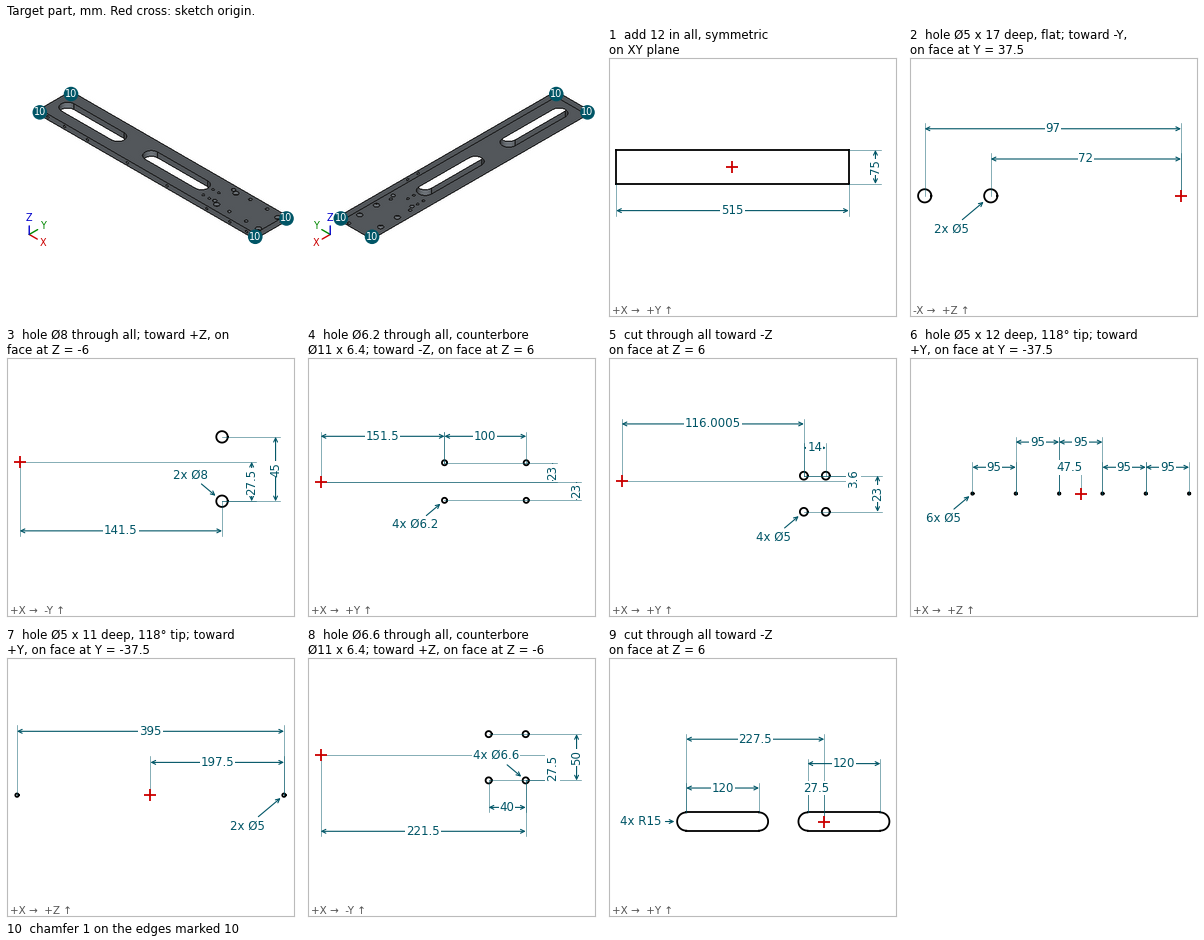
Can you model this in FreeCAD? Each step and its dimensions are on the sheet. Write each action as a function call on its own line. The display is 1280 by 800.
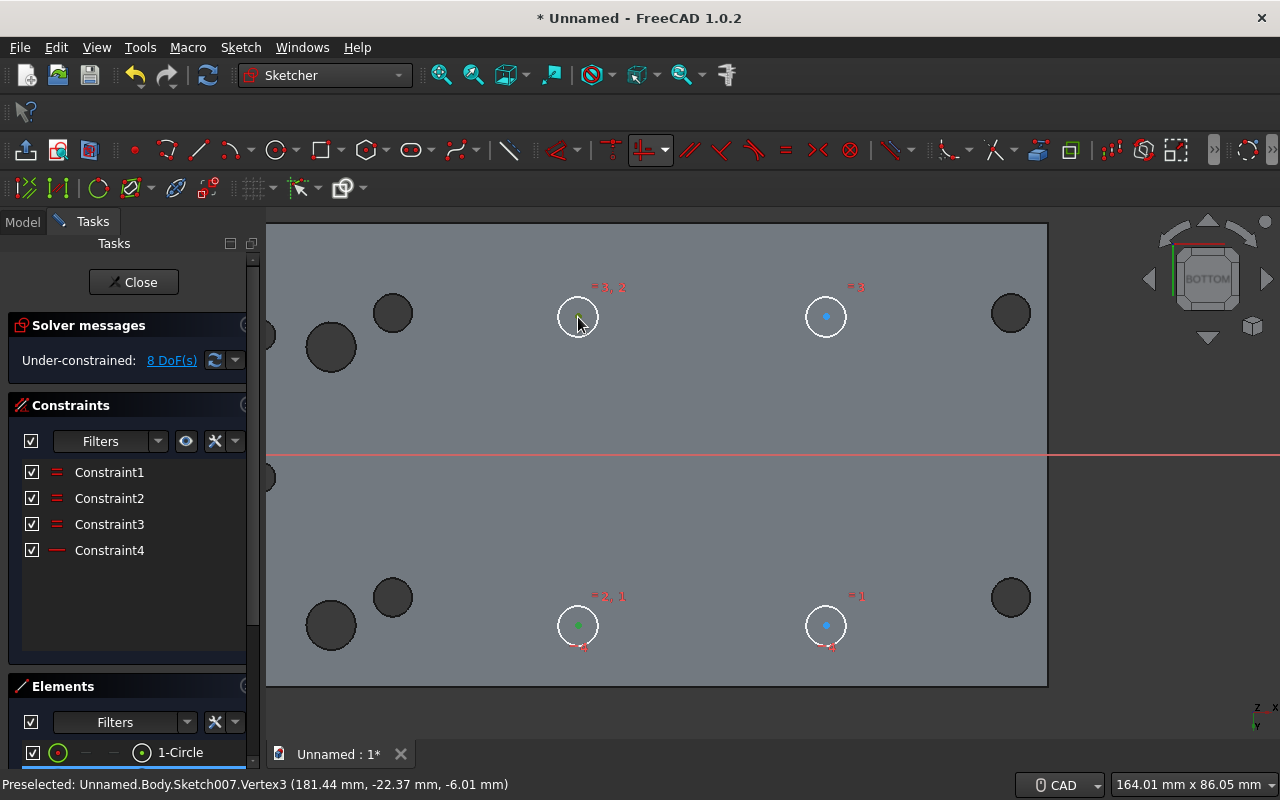
key(v)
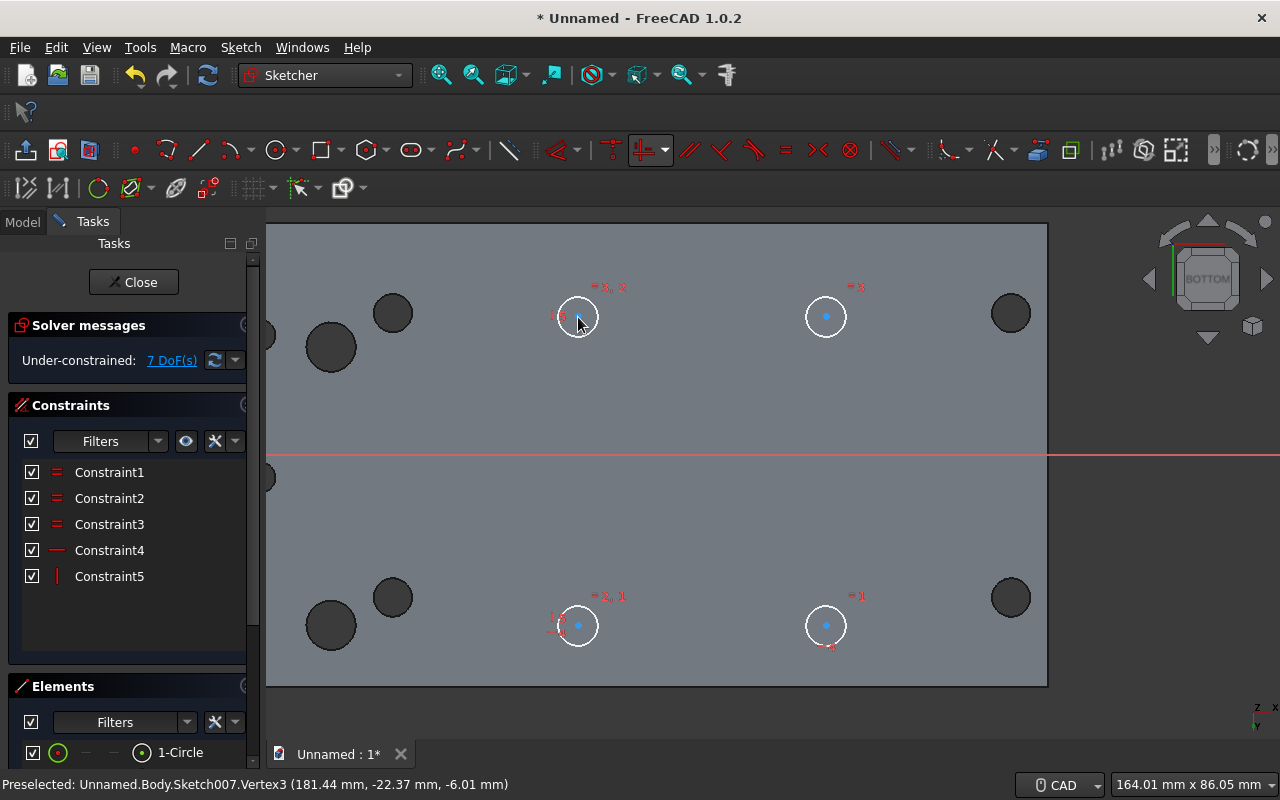
click(826, 626)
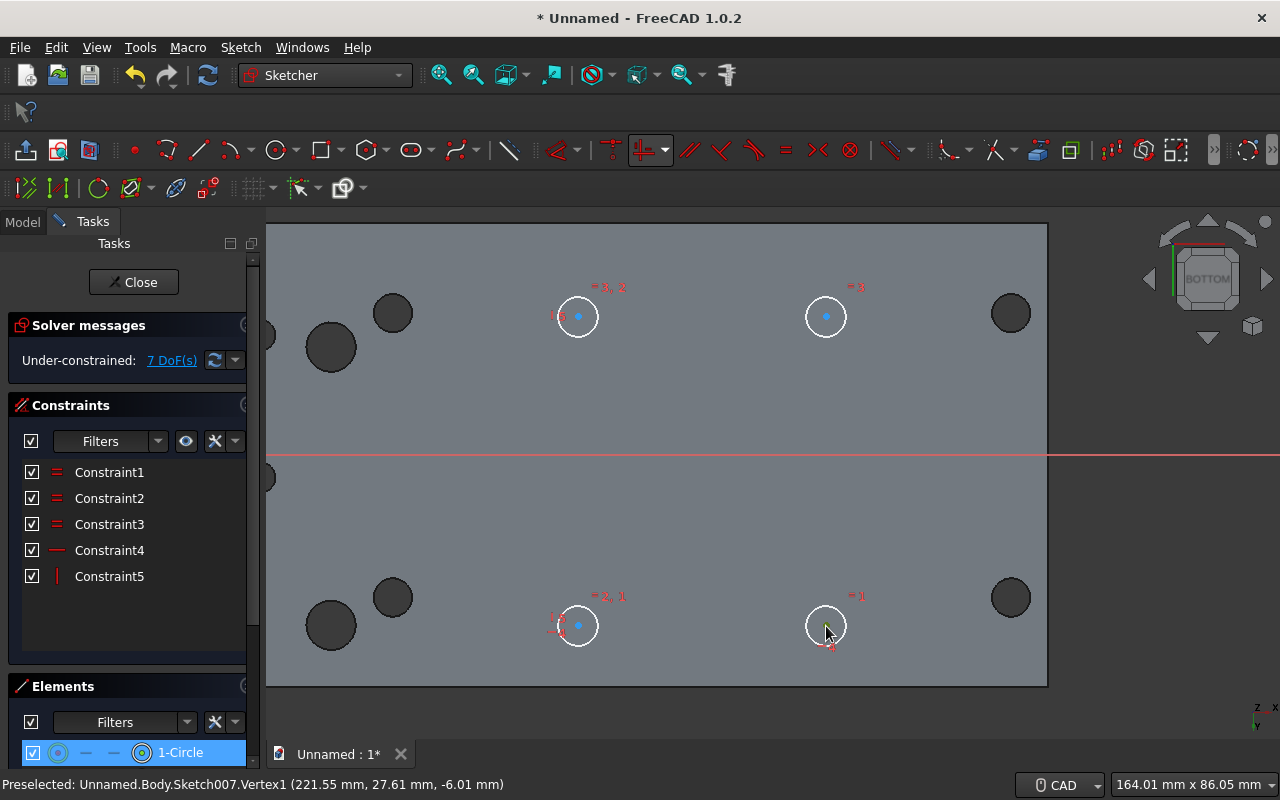
click(826, 317)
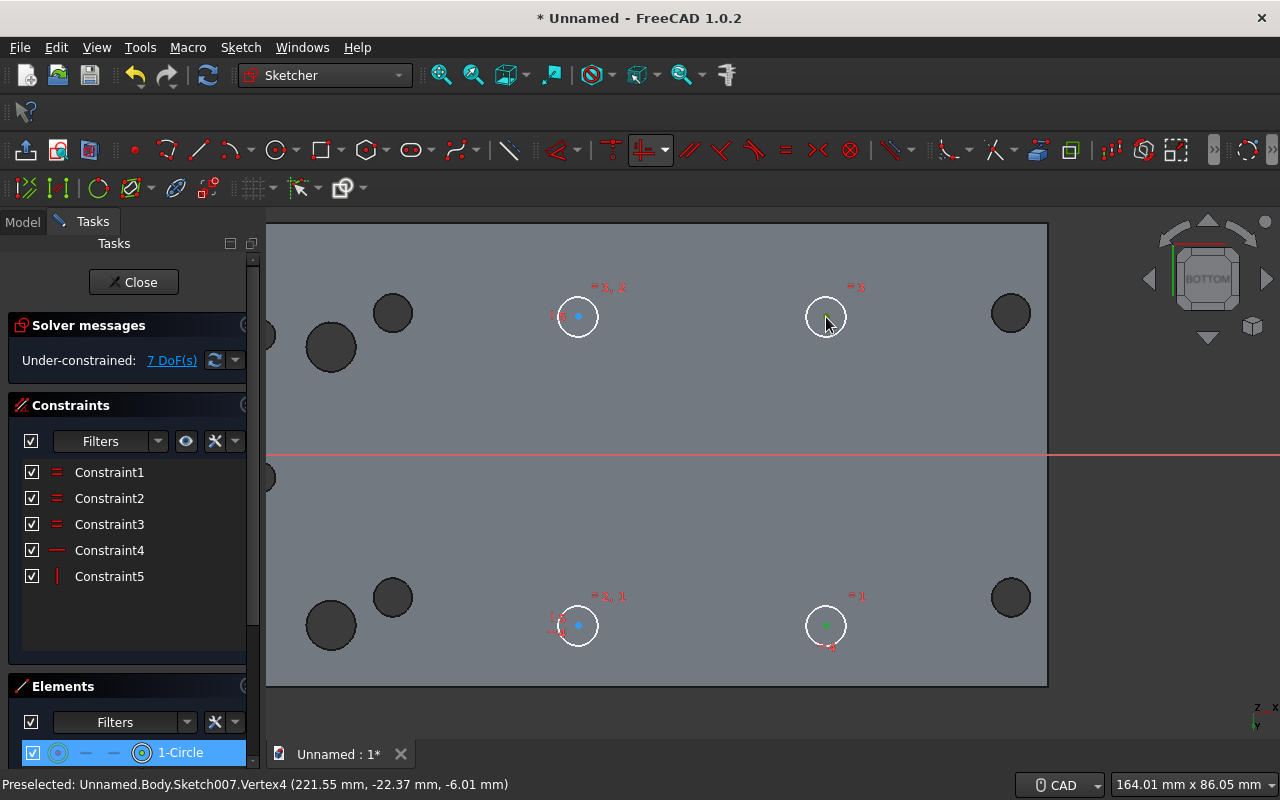
key(v)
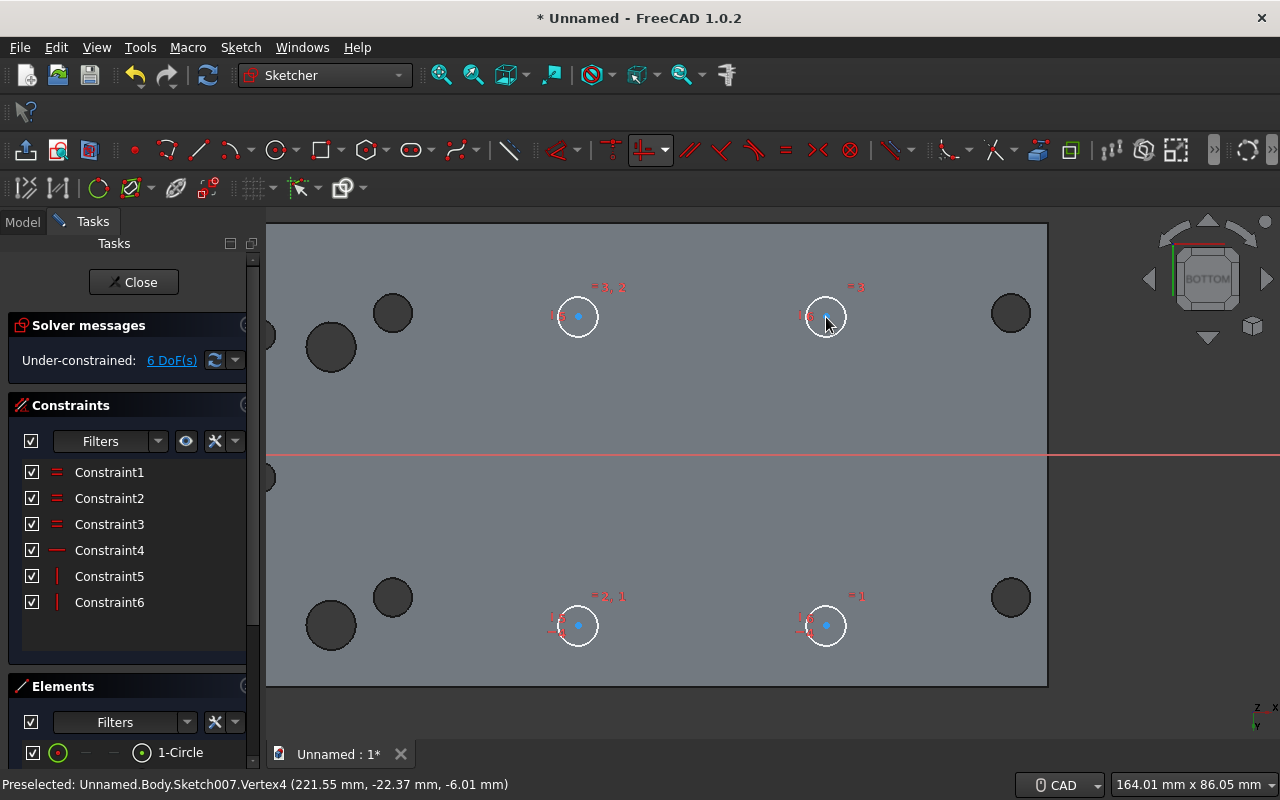
click(578, 317)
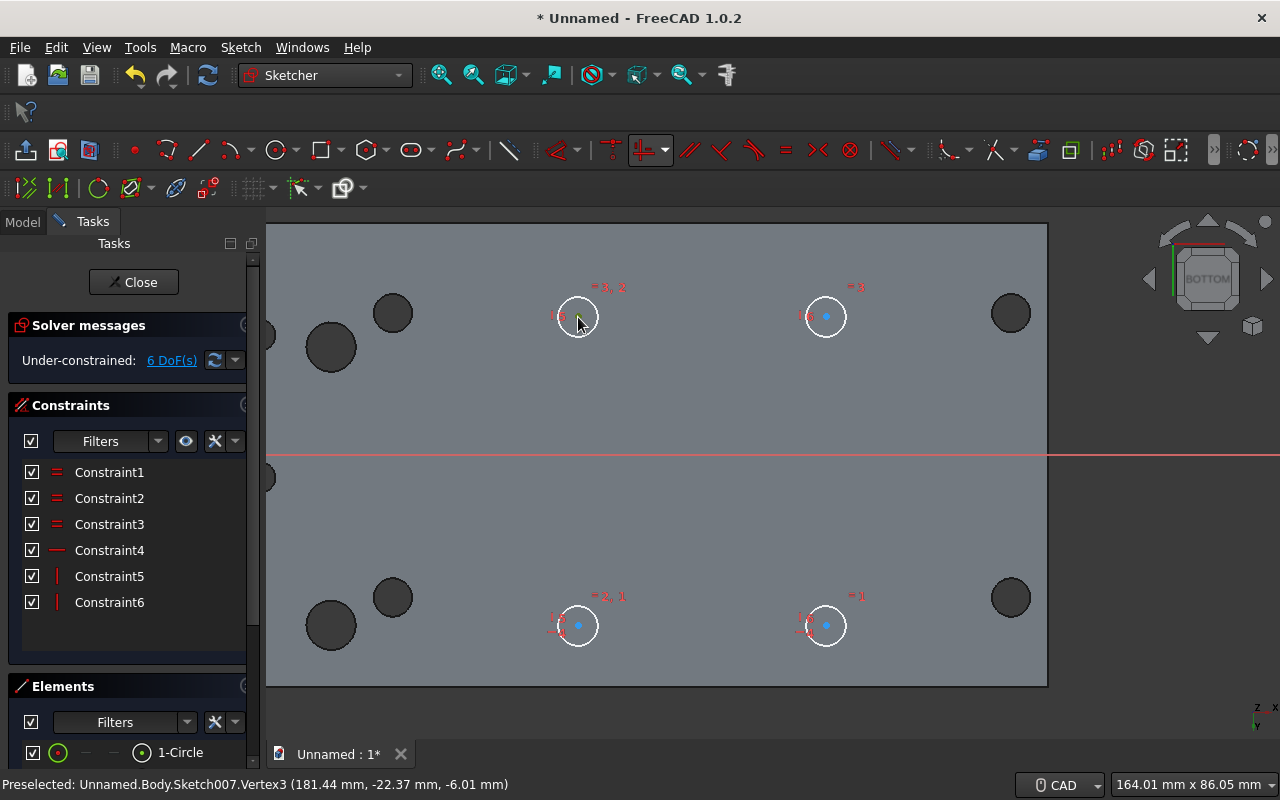
click(826, 317)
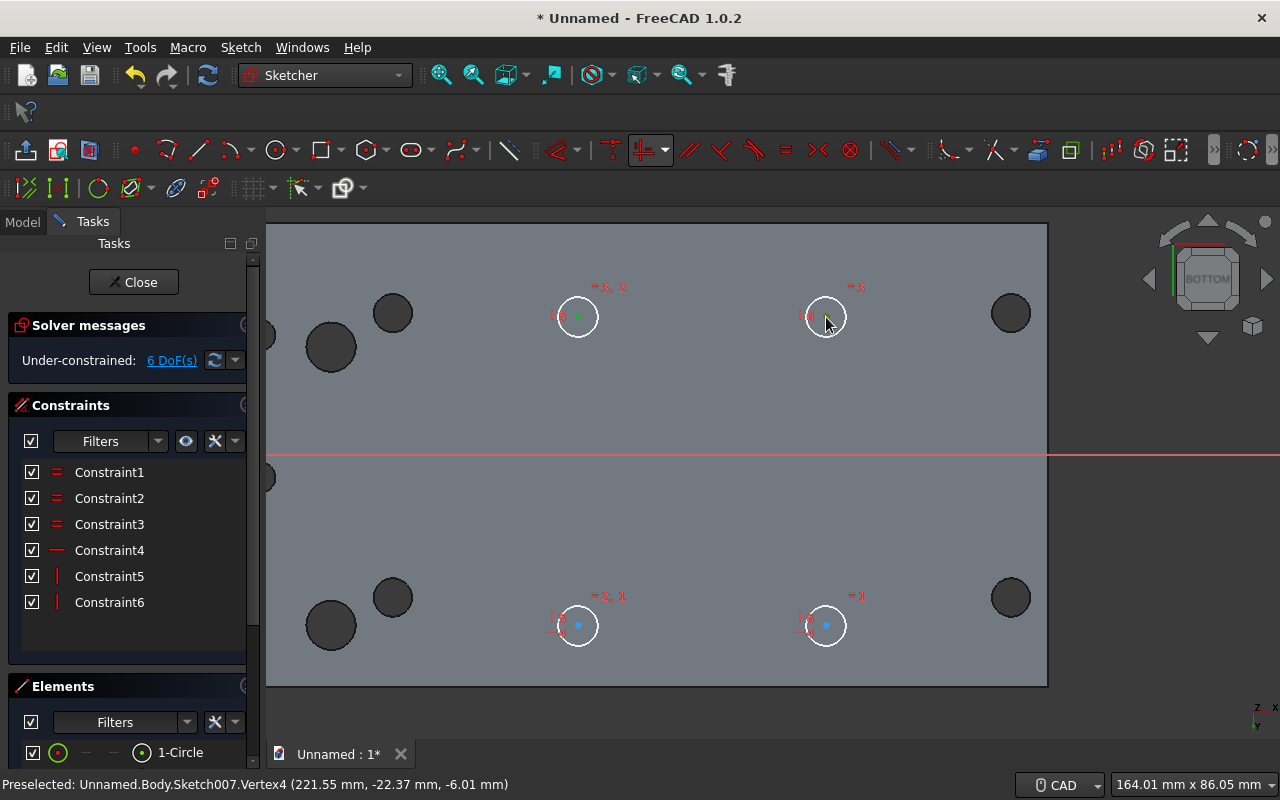
click(668, 150)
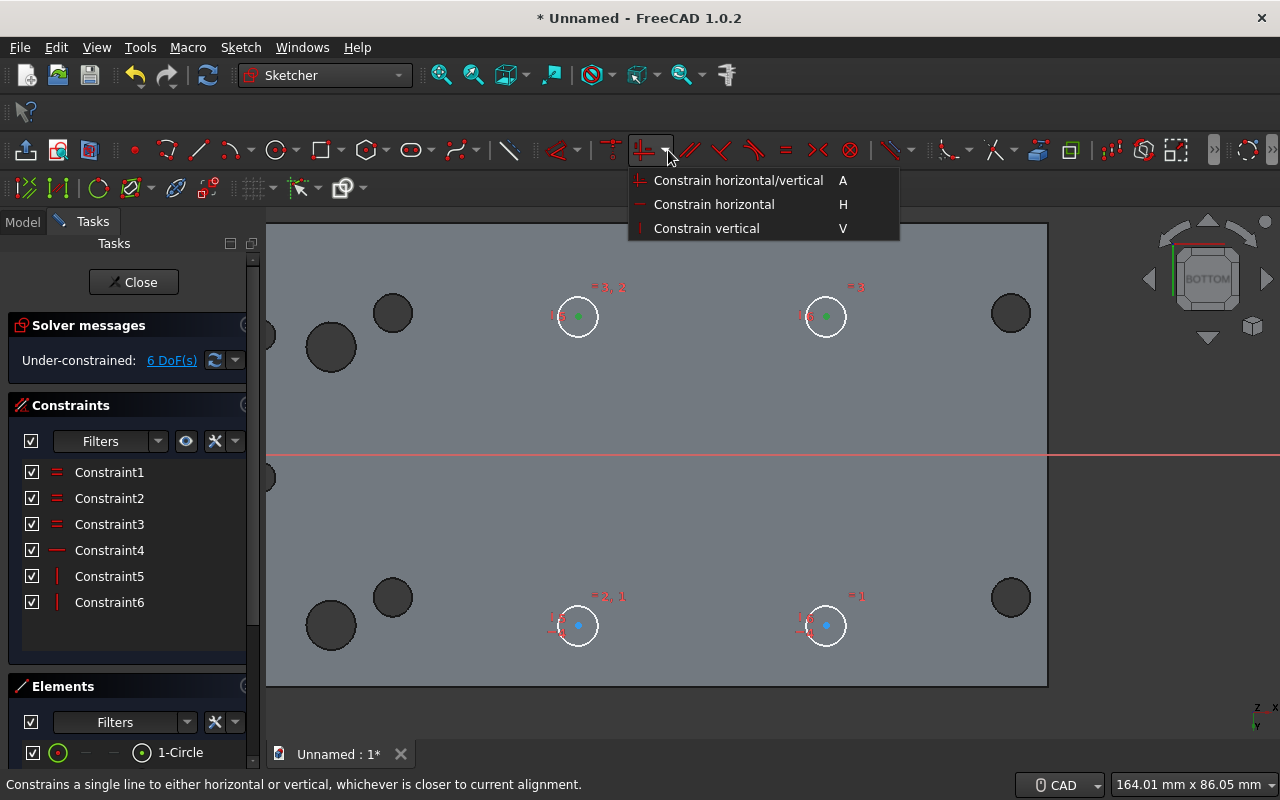
click(764, 204)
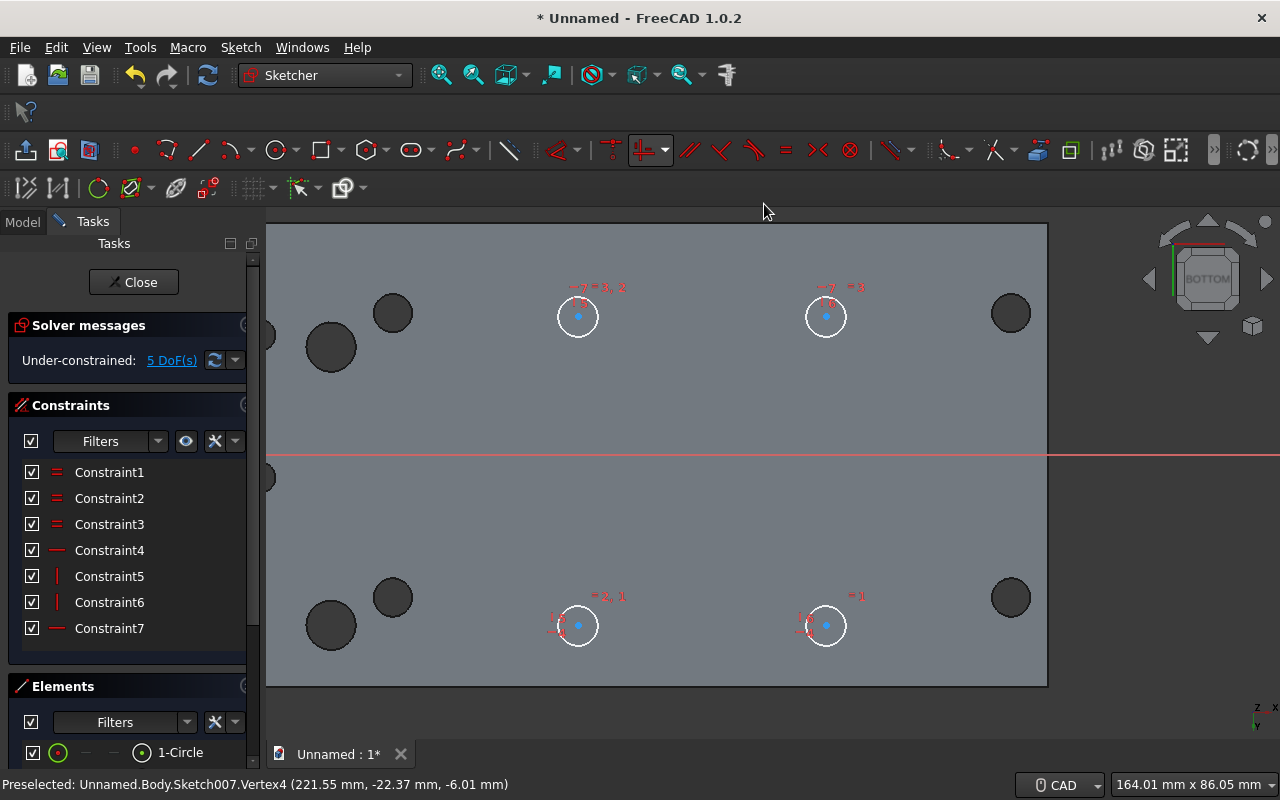
key(d)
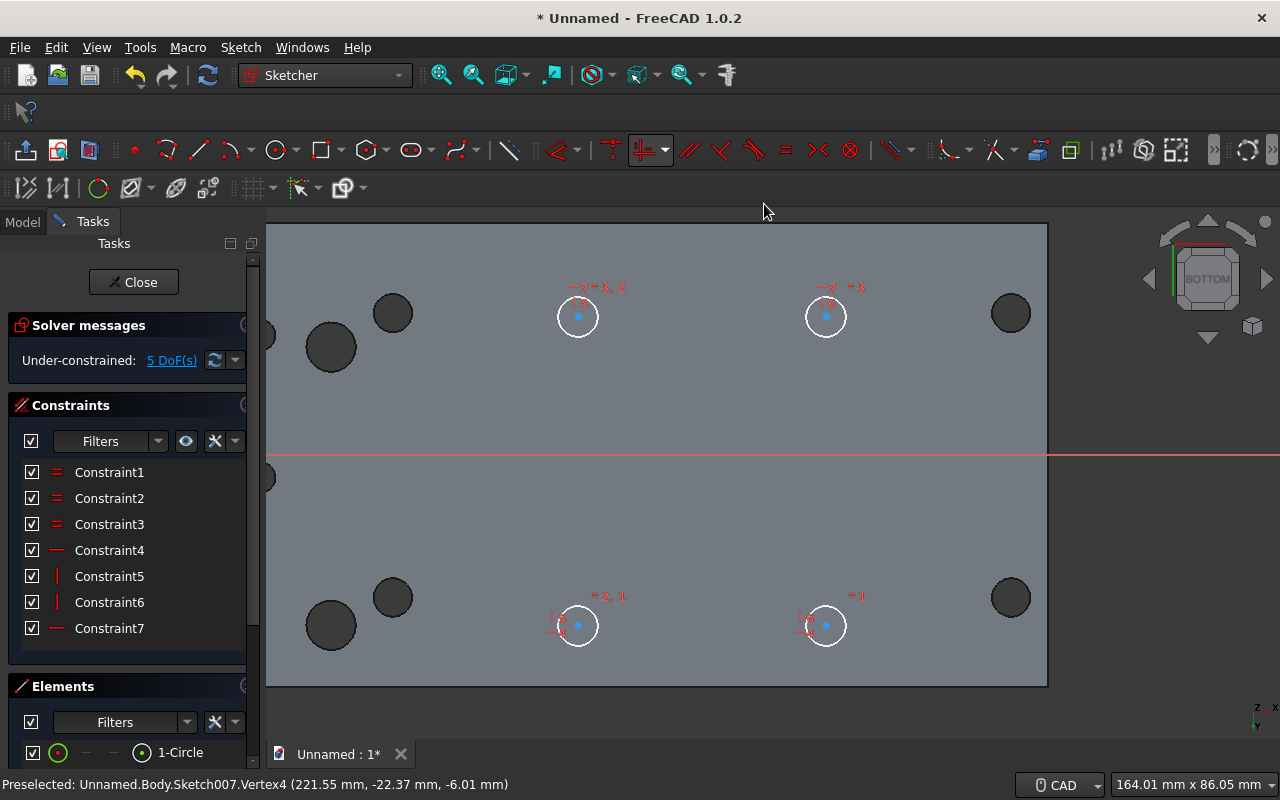
click(840, 612)
click(863, 589)